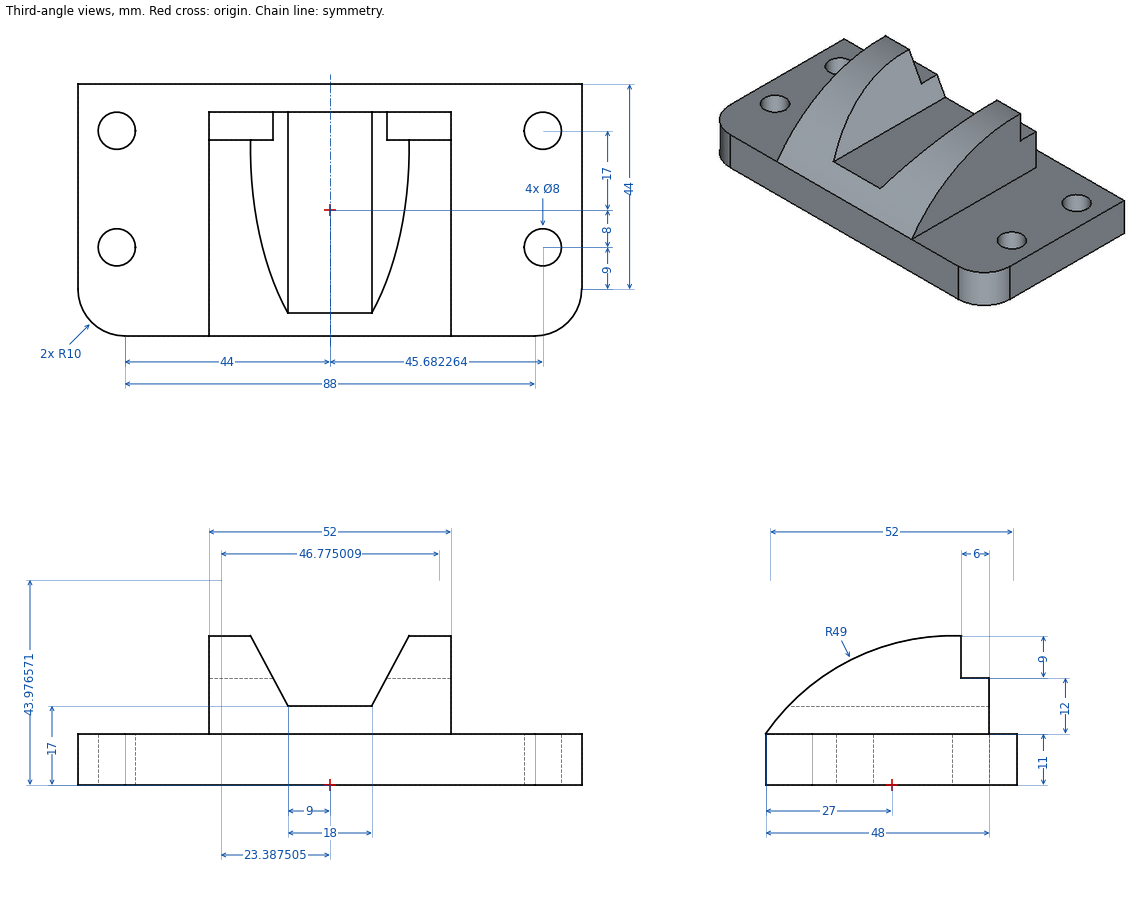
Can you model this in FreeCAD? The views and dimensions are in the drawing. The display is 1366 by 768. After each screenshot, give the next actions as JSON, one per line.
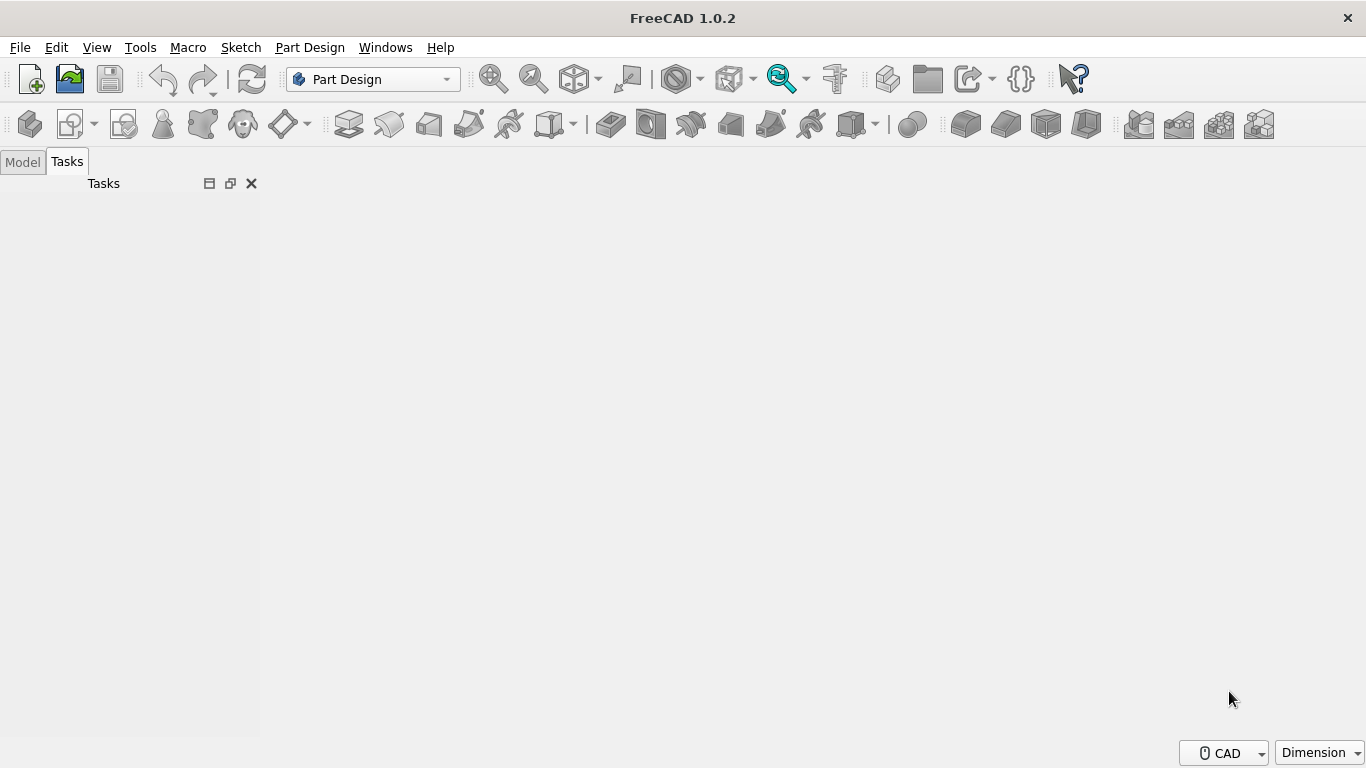
{"action": "left_click", "coordinate": [30, 80]}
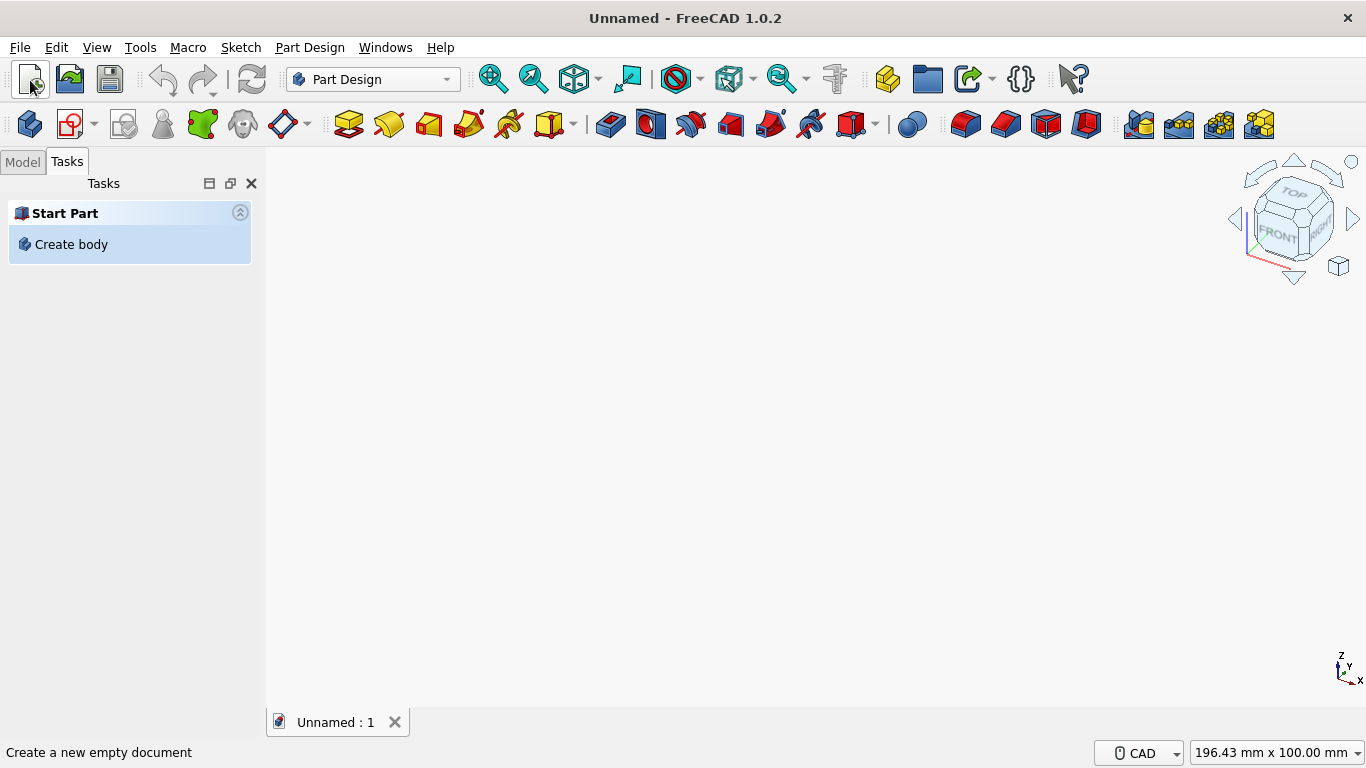
{"action": "left_click", "coordinate": [70, 124]}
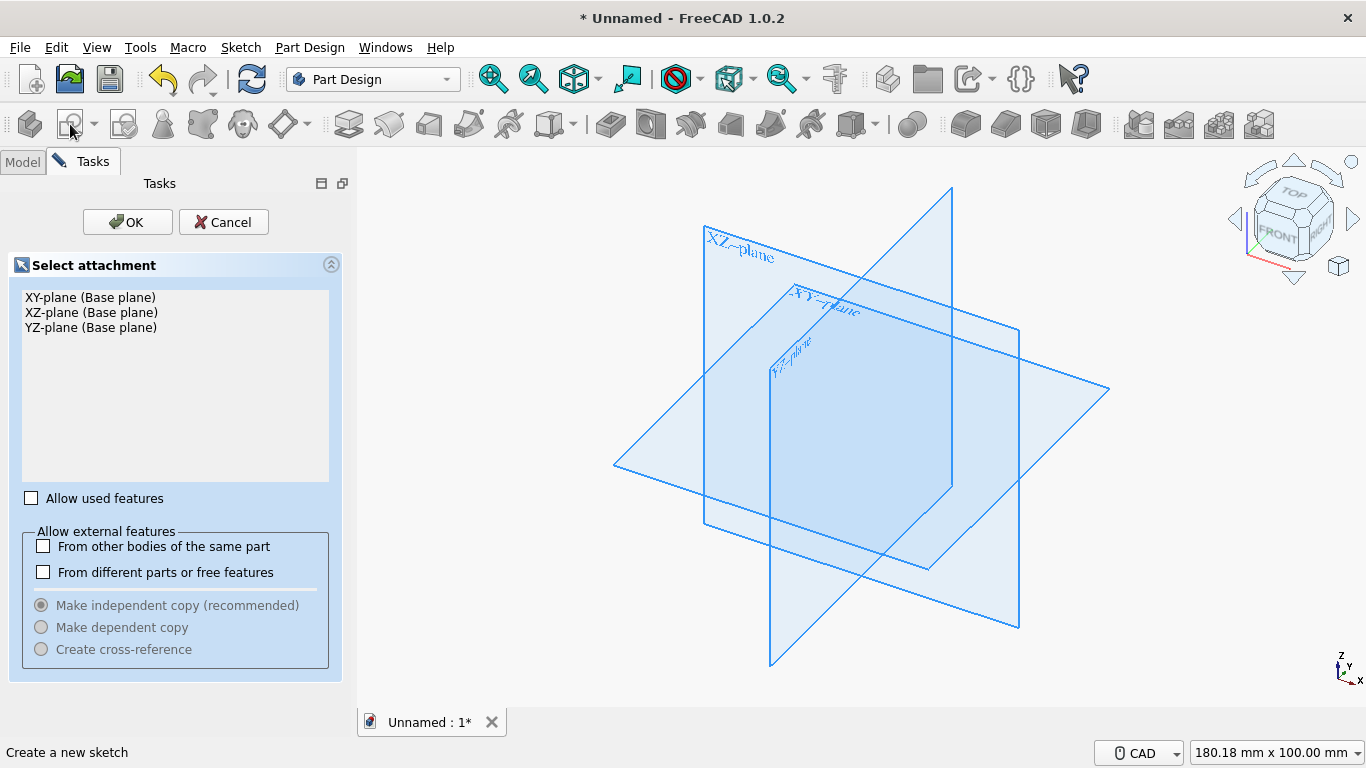
{"action": "left_click", "coordinate": [82, 298]}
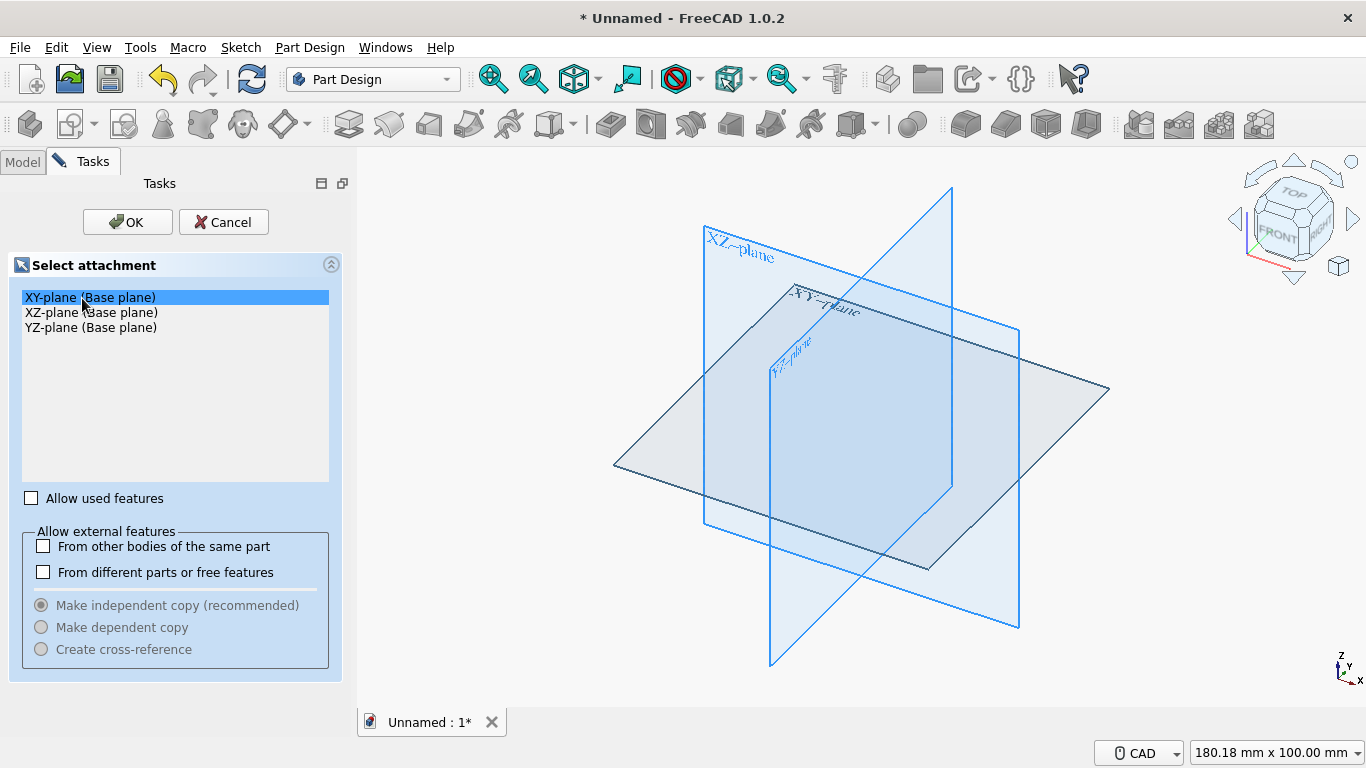
{"action": "left_click", "coordinate": [128, 222]}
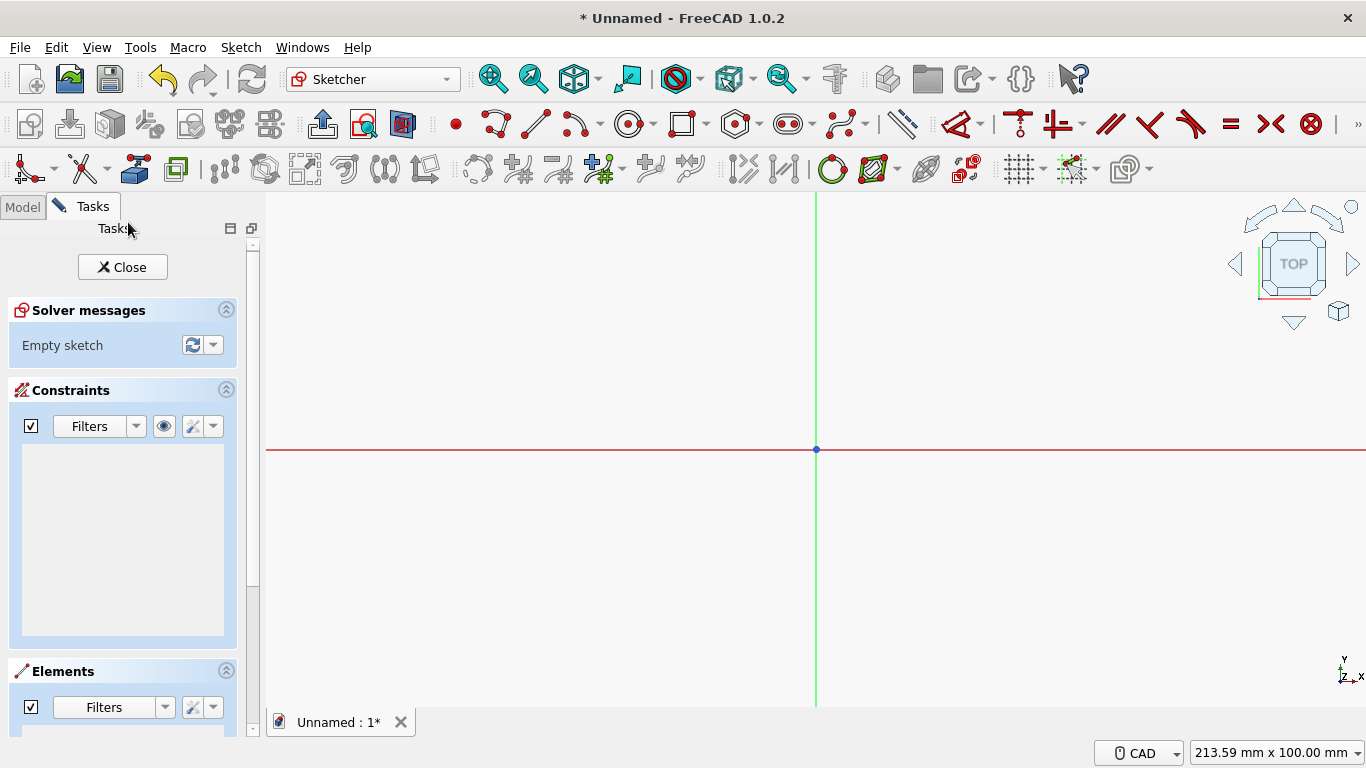
{"action": "key", "text": "g l"}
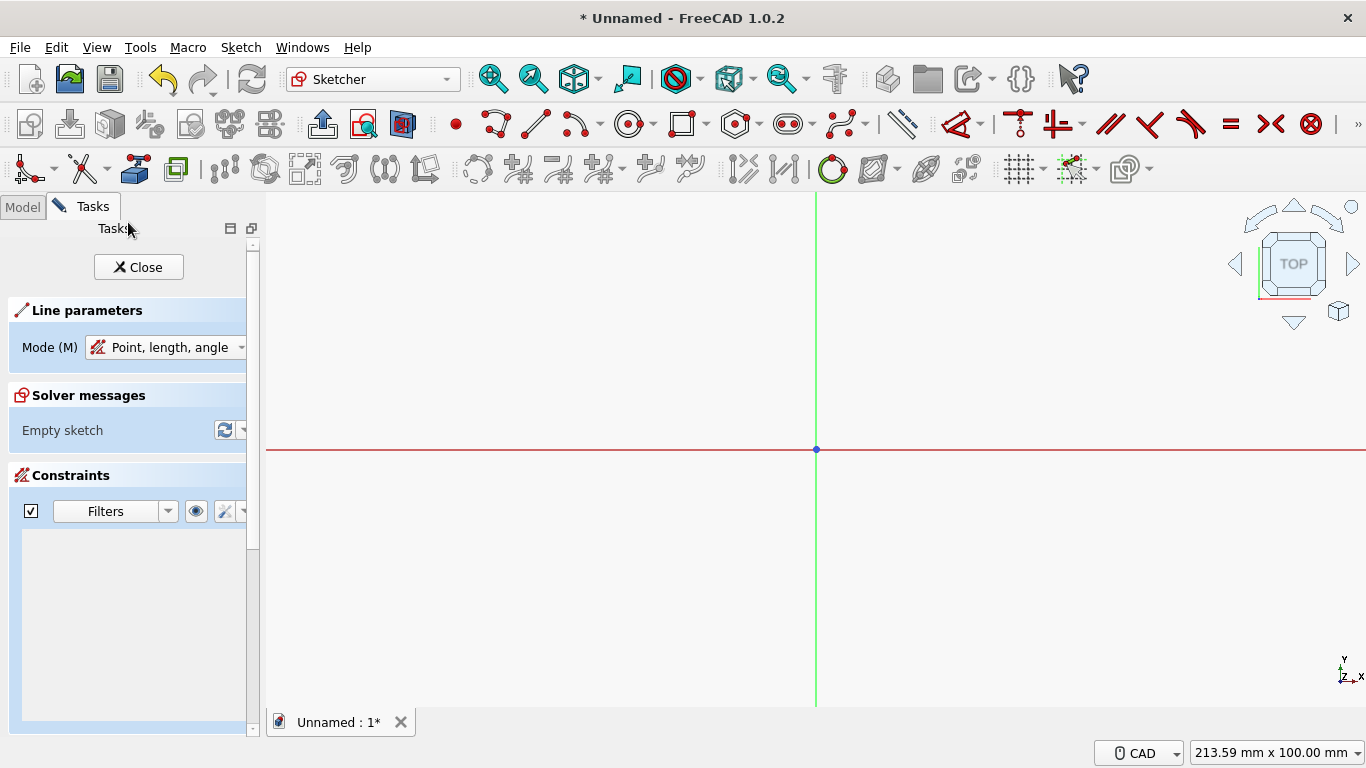
{"action": "left_click", "coordinate": [589, 589]}
{"action": "left_click", "coordinate": [1043, 589]}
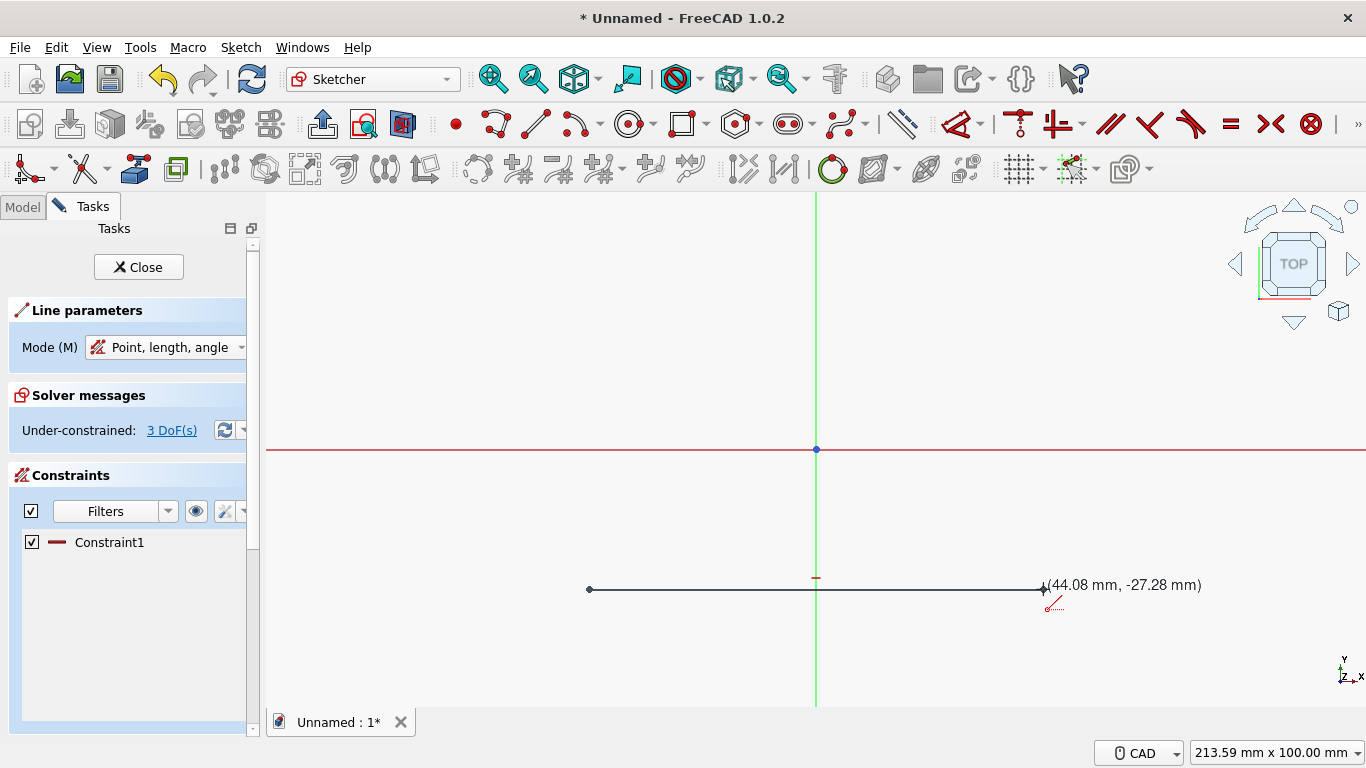
{"action": "key", "text": "g m"}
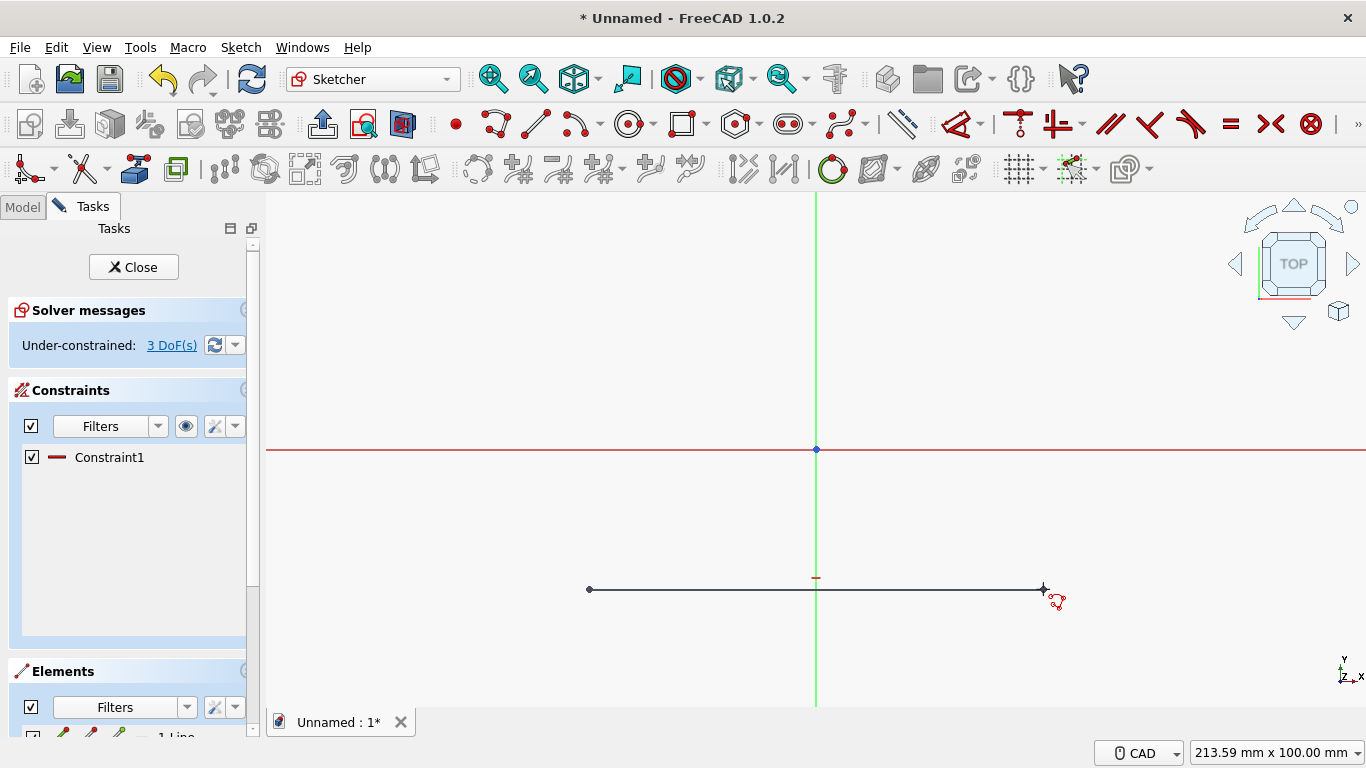
{"action": "left_click", "coordinate": [1094, 537]}
{"action": "left_click", "coordinate": [1094, 310]}
{"action": "left_click", "coordinate": [538, 310]}
{"action": "left_click", "coordinate": [538, 537]}
{"action": "right_click", "coordinate": [538, 537]}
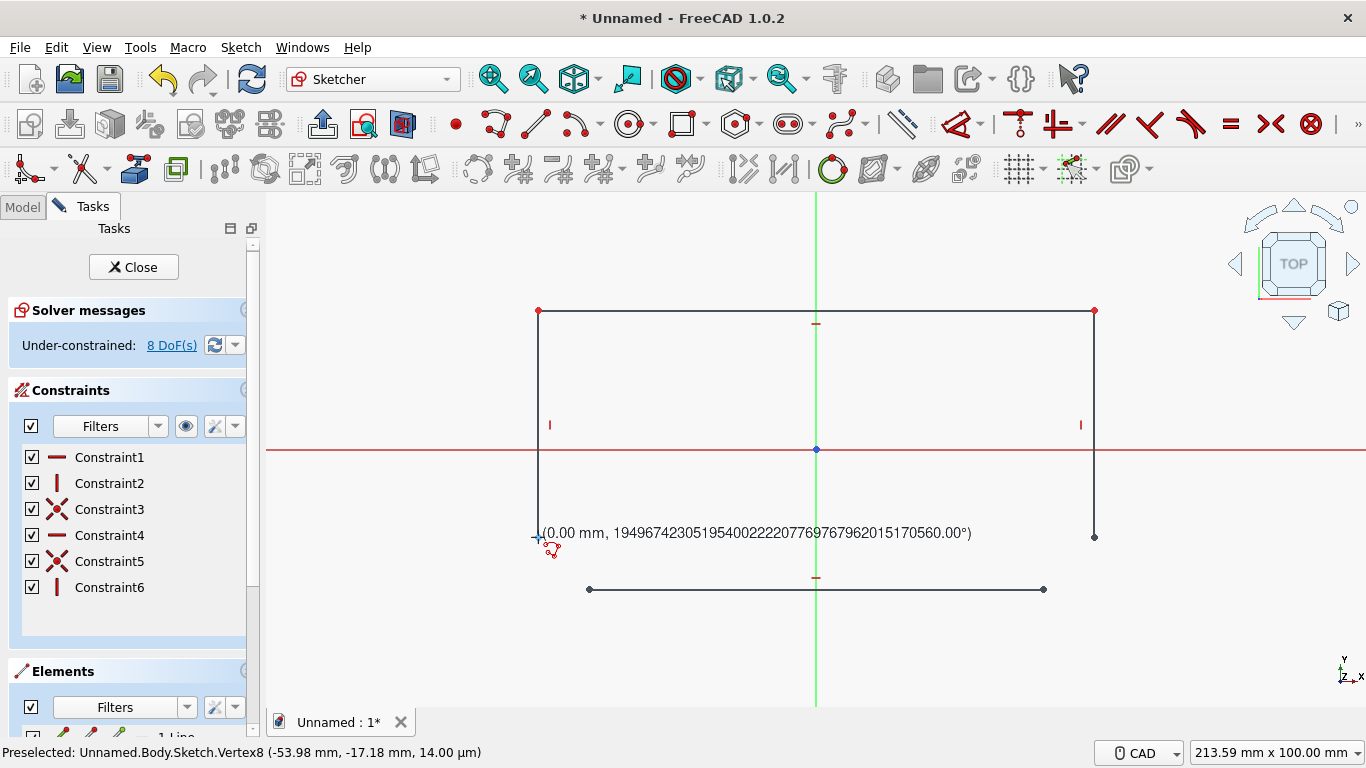
{"action": "key", "text": "g 3 a"}